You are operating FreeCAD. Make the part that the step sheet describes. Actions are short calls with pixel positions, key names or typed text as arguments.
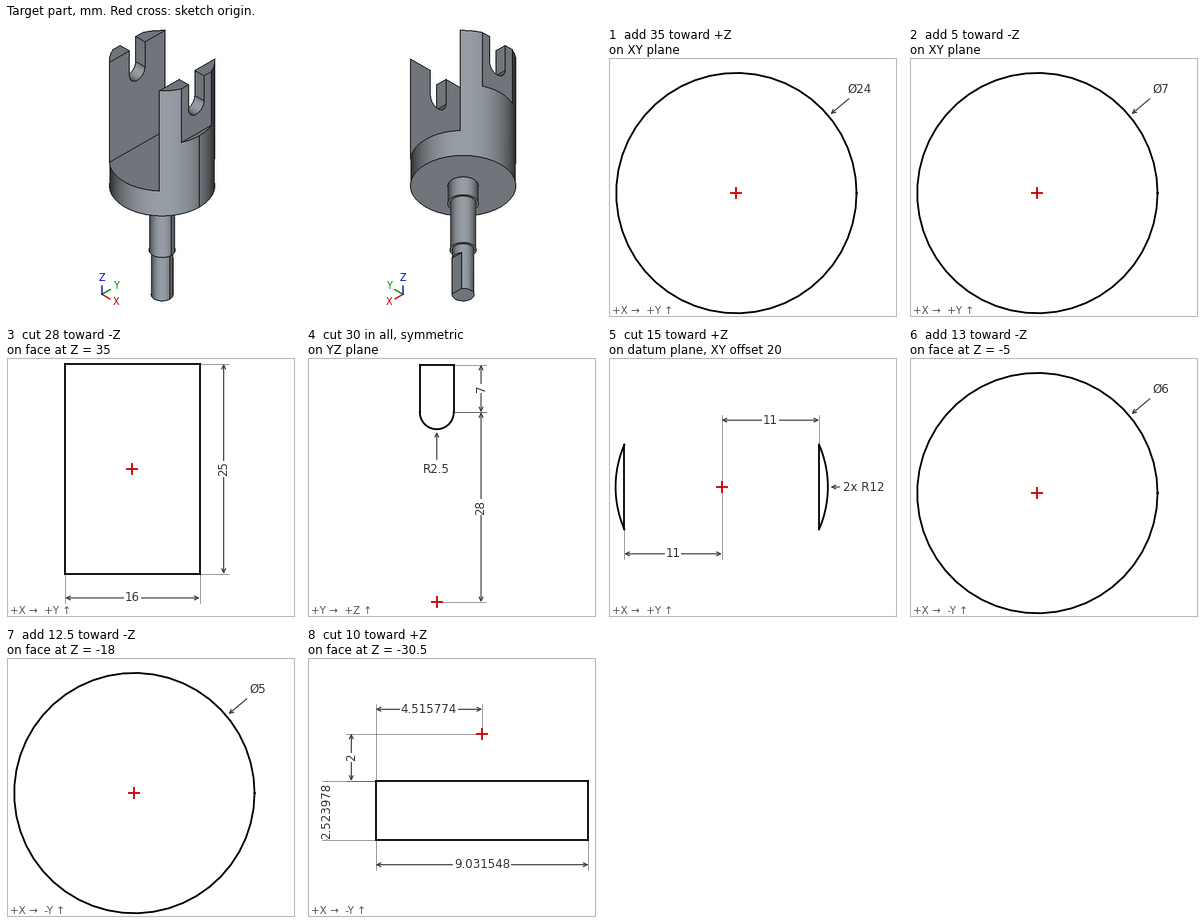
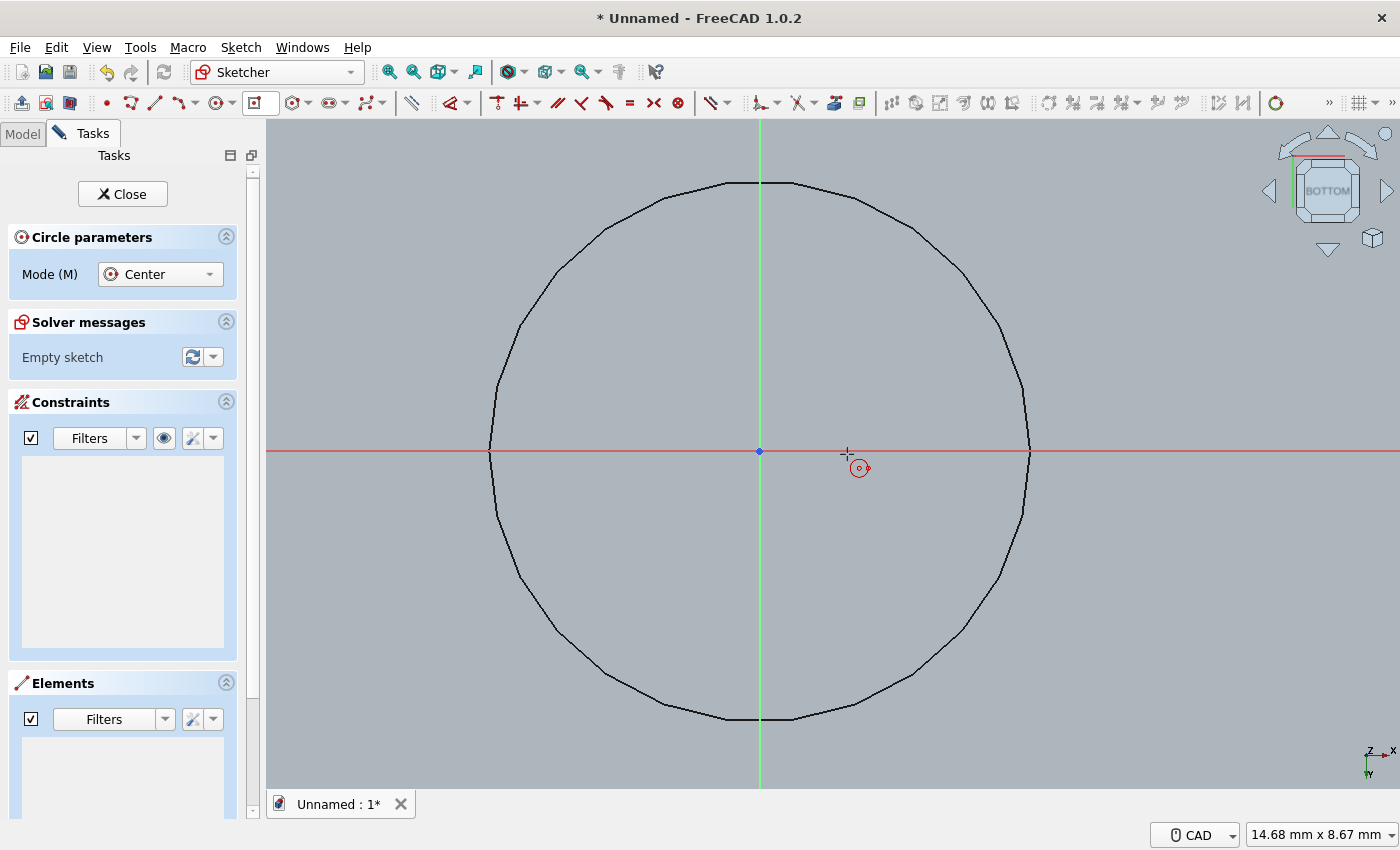
click(760, 451)
click(924, 288)
key(Escape)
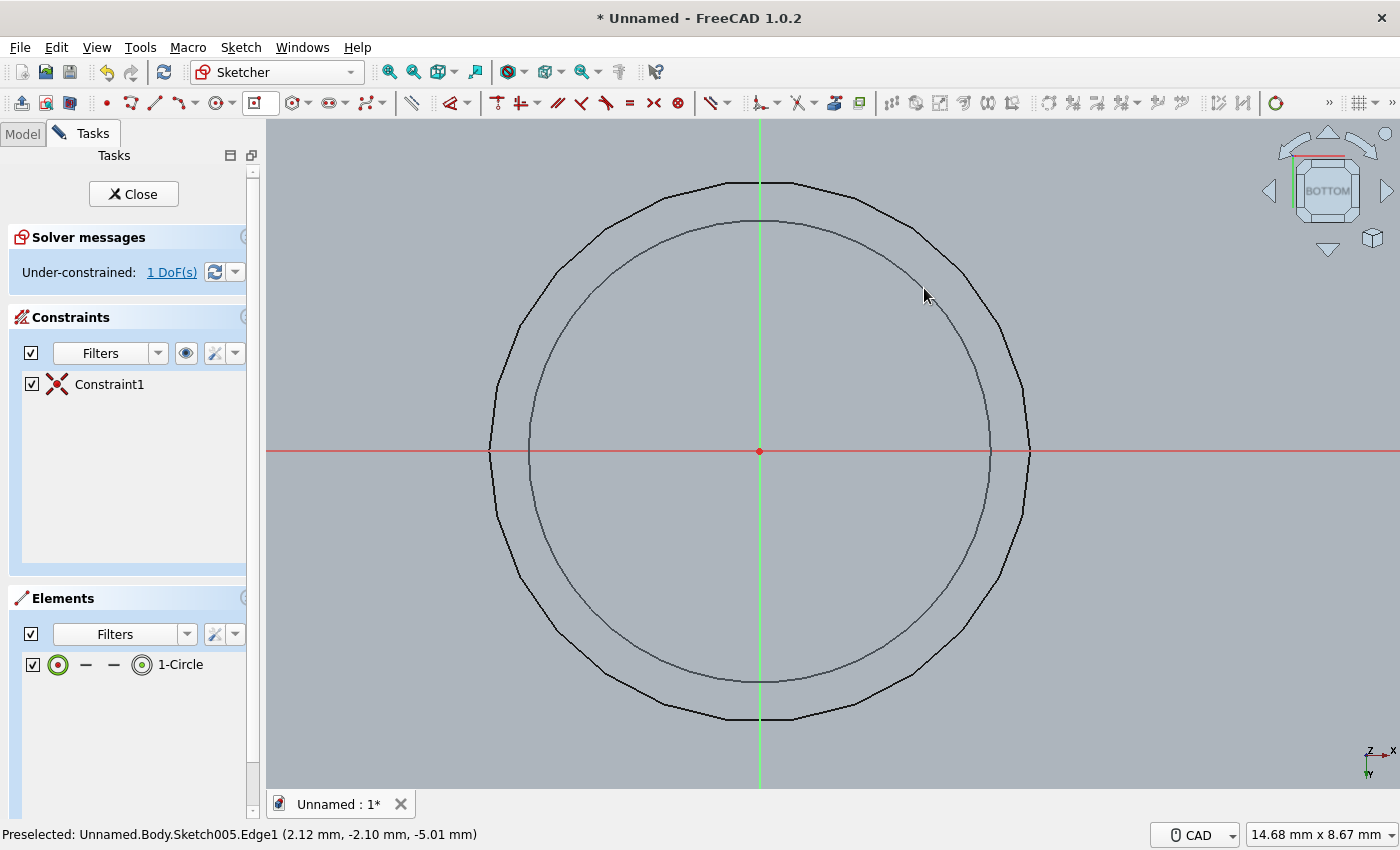
key(d)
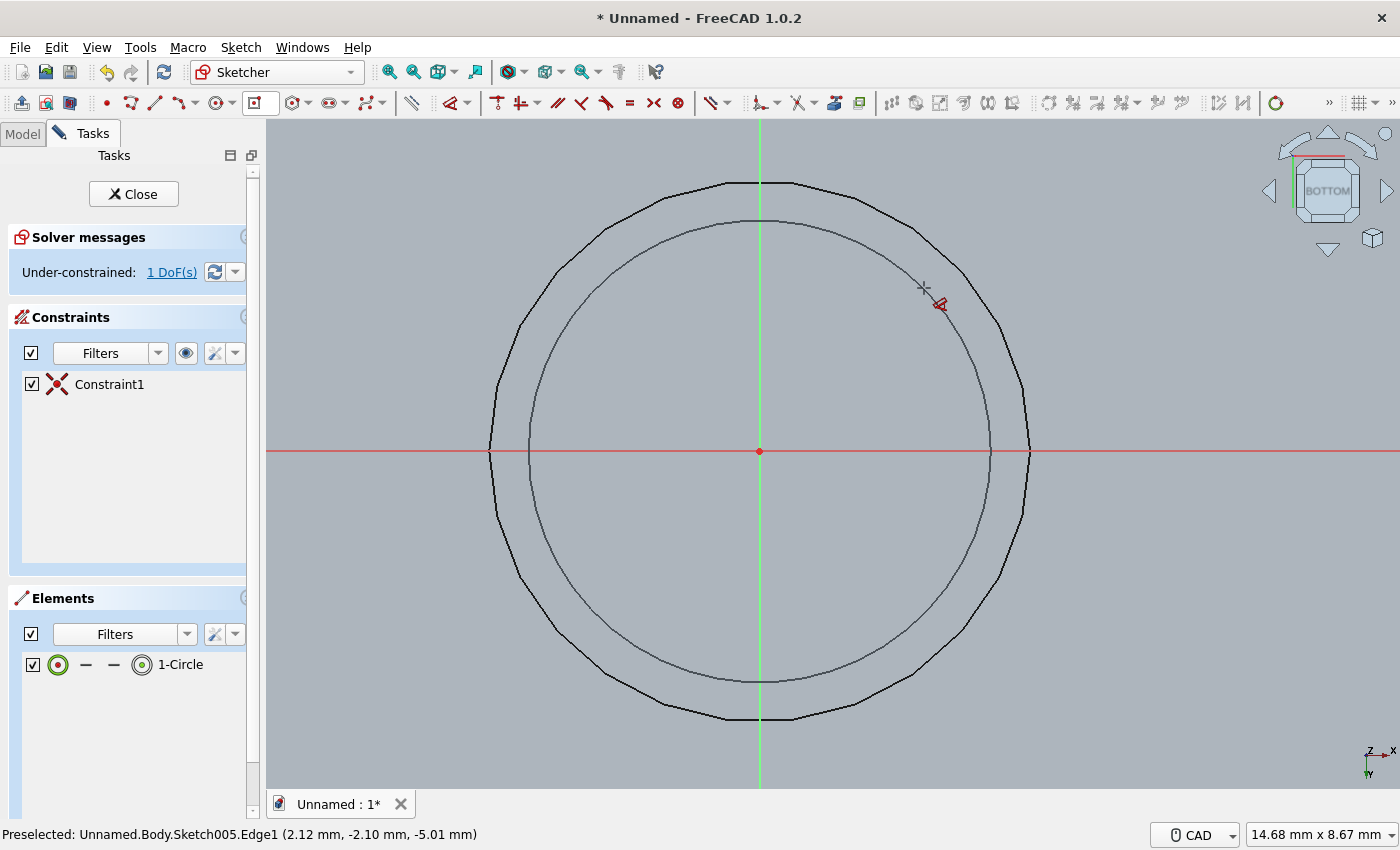
click(923, 288)
click(946, 265)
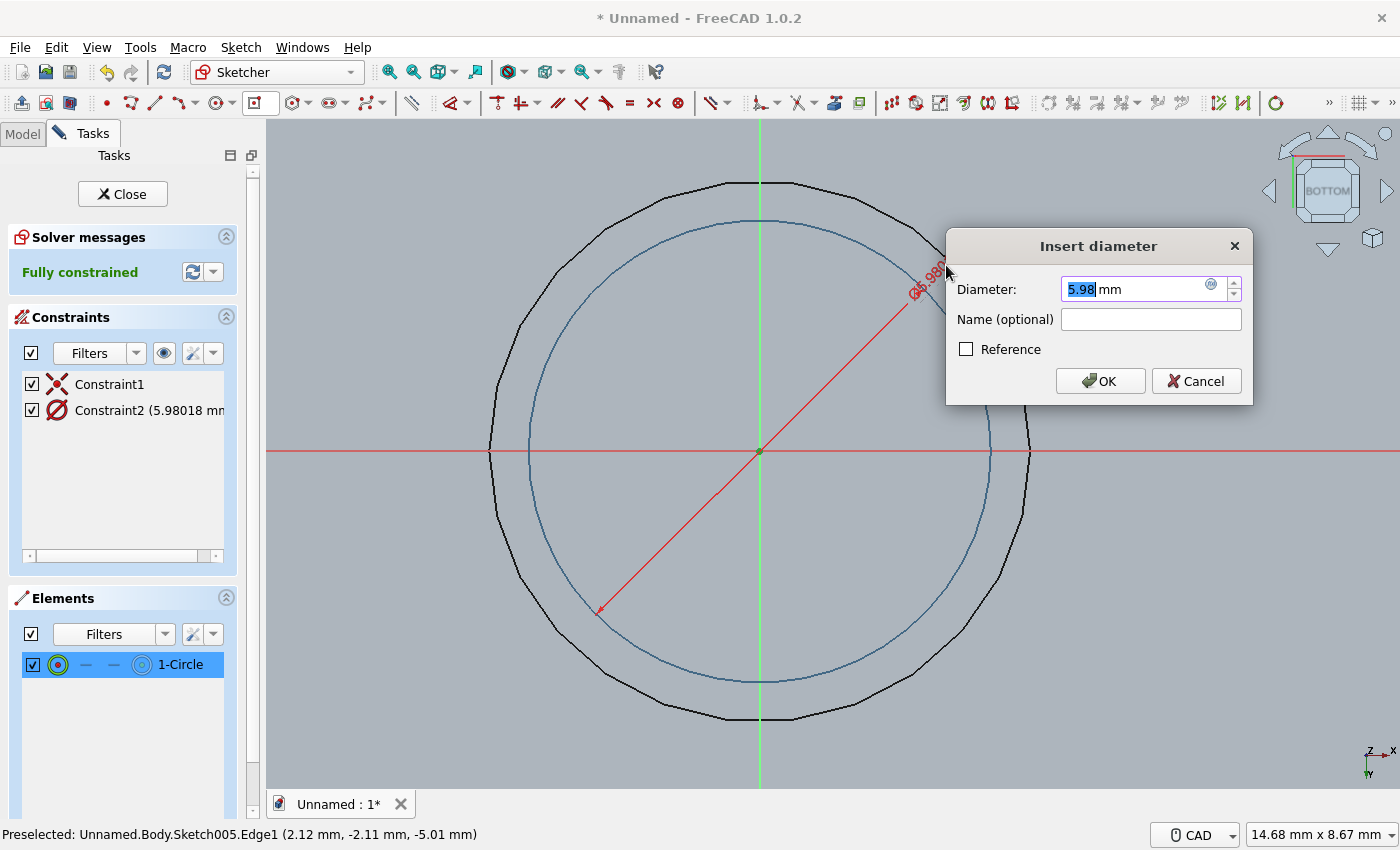
text(6)
key(Return)
key(Escape)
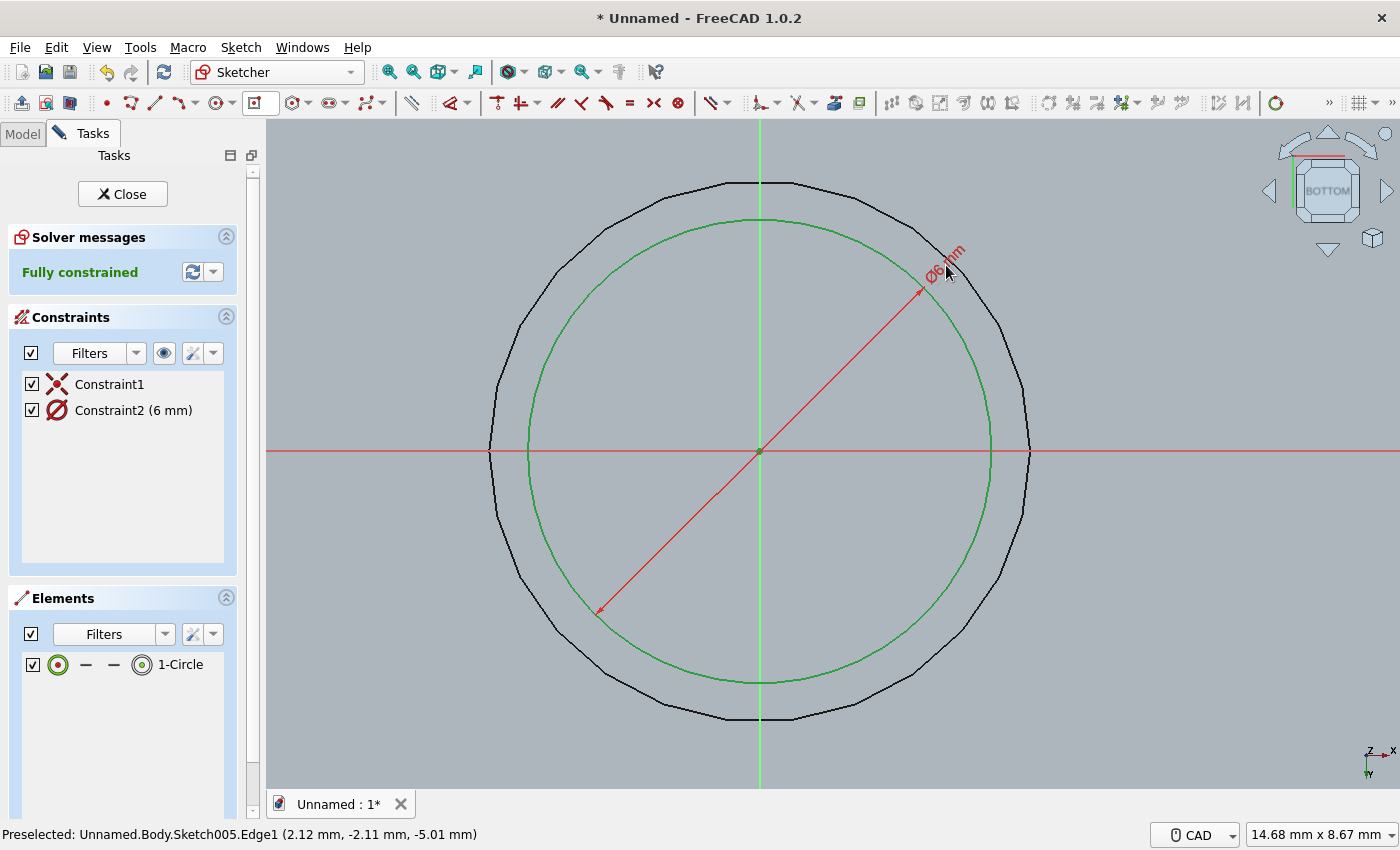
click(123, 194)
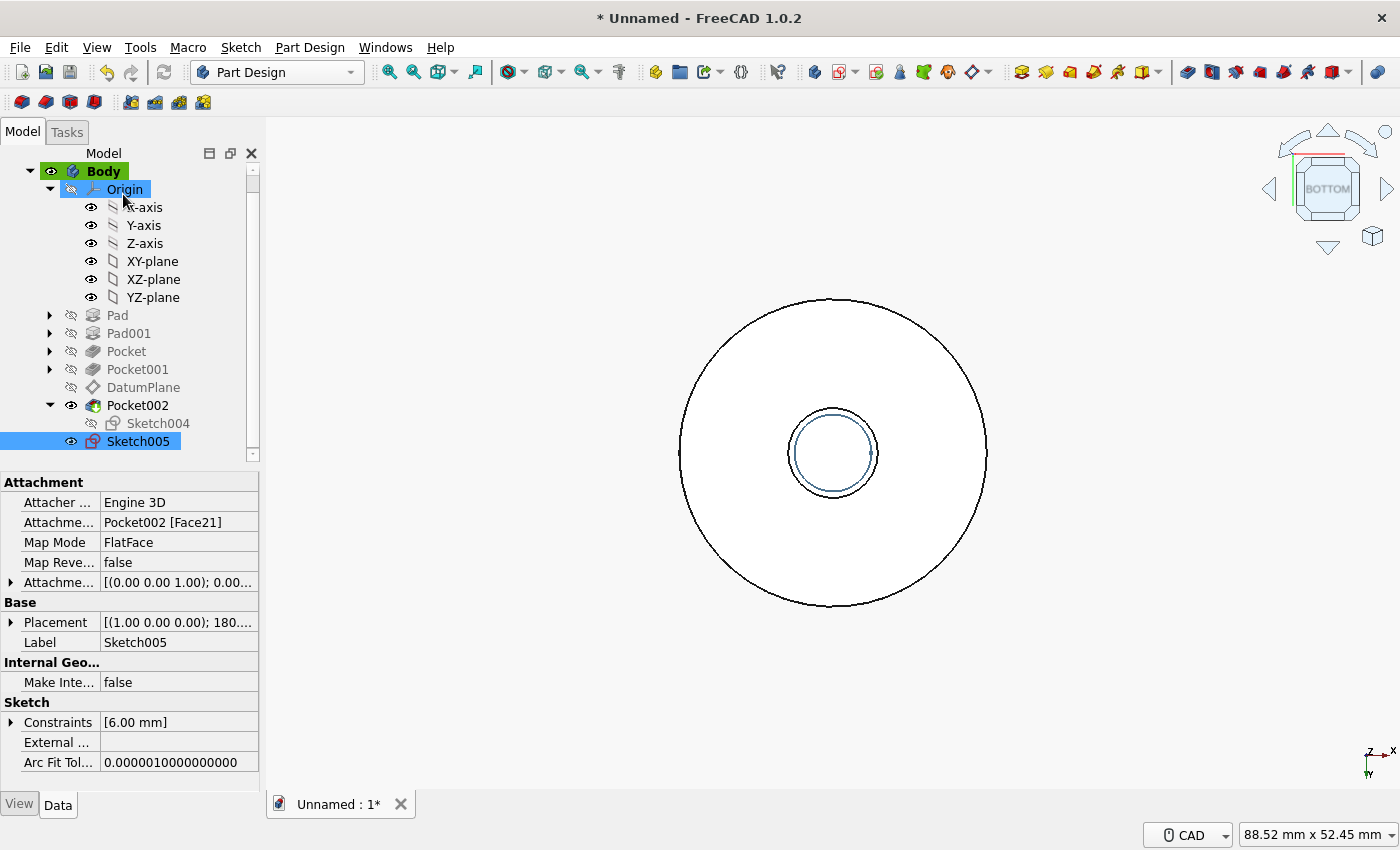
click(1022, 72)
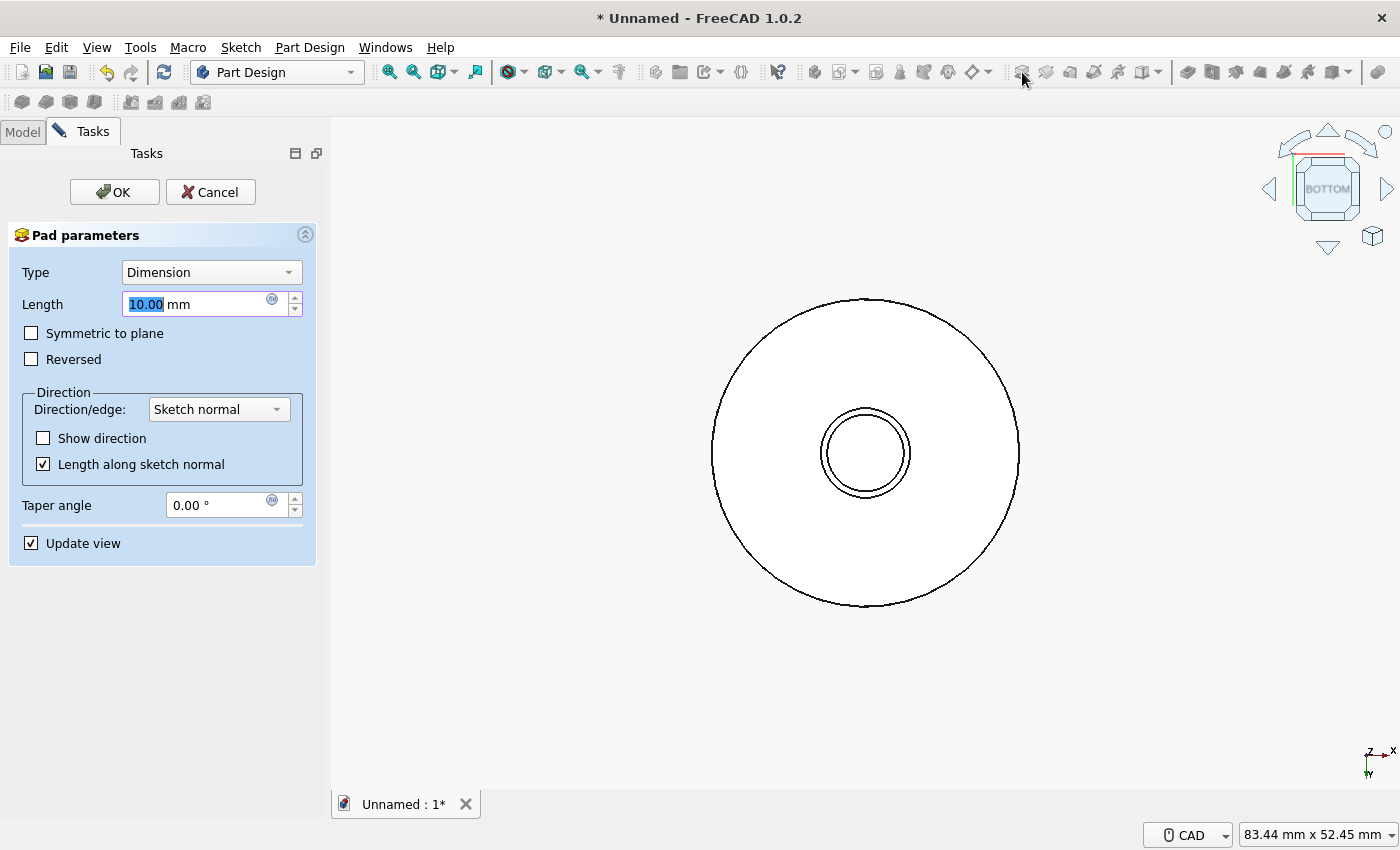
text(13)
key(Tab)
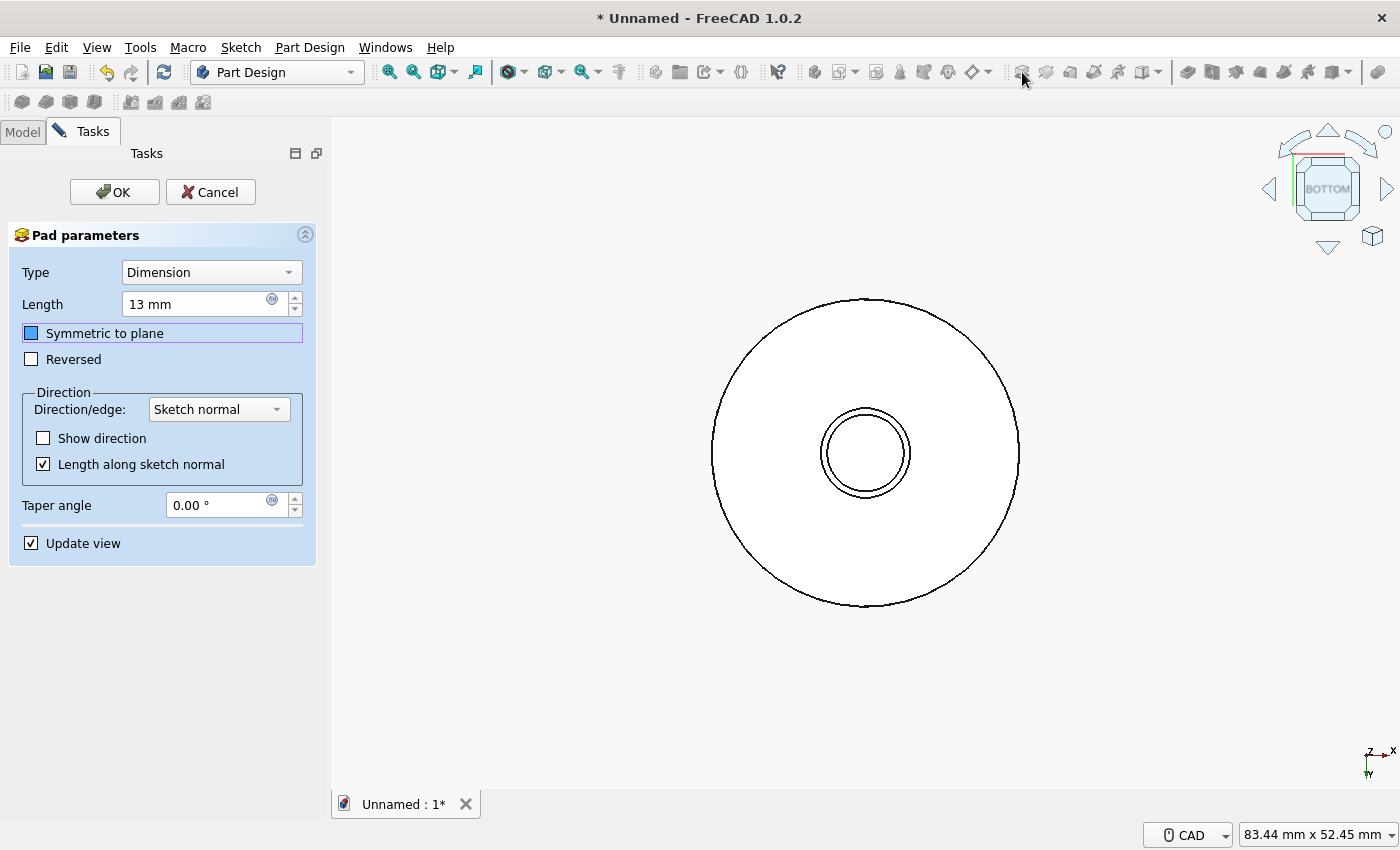
click(115, 192)